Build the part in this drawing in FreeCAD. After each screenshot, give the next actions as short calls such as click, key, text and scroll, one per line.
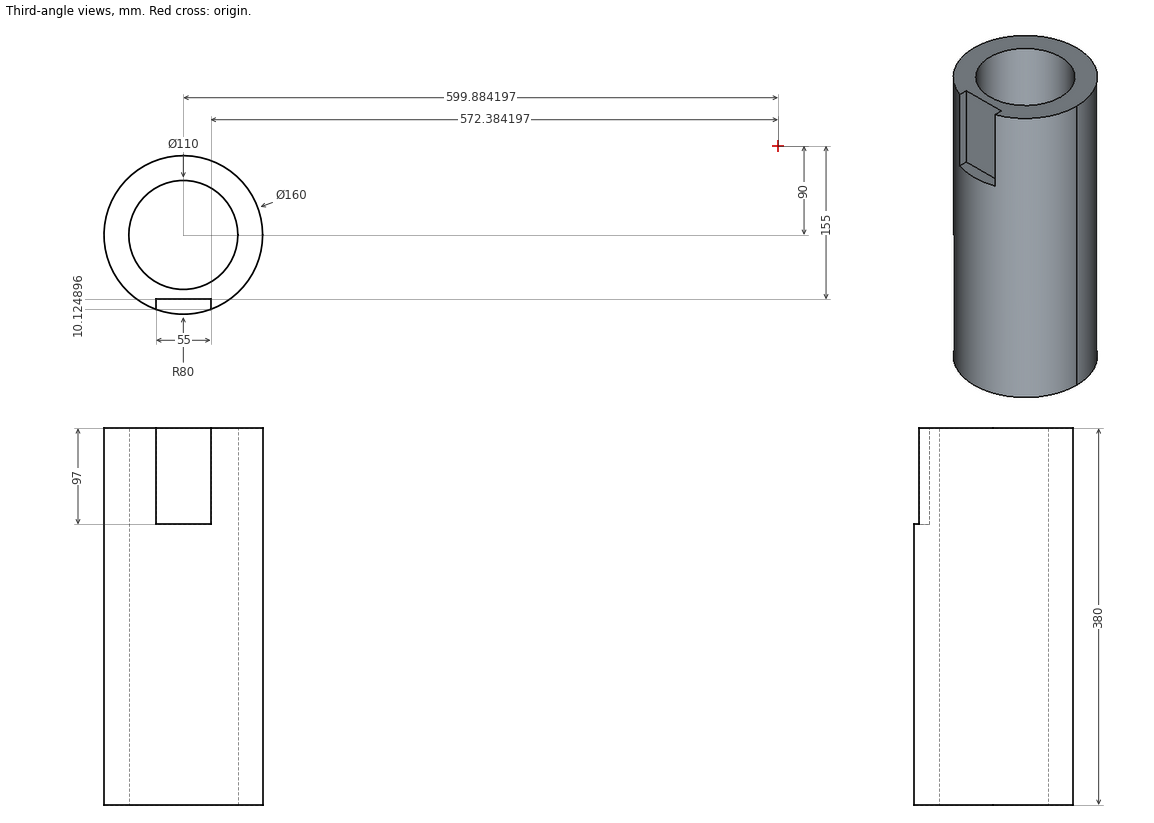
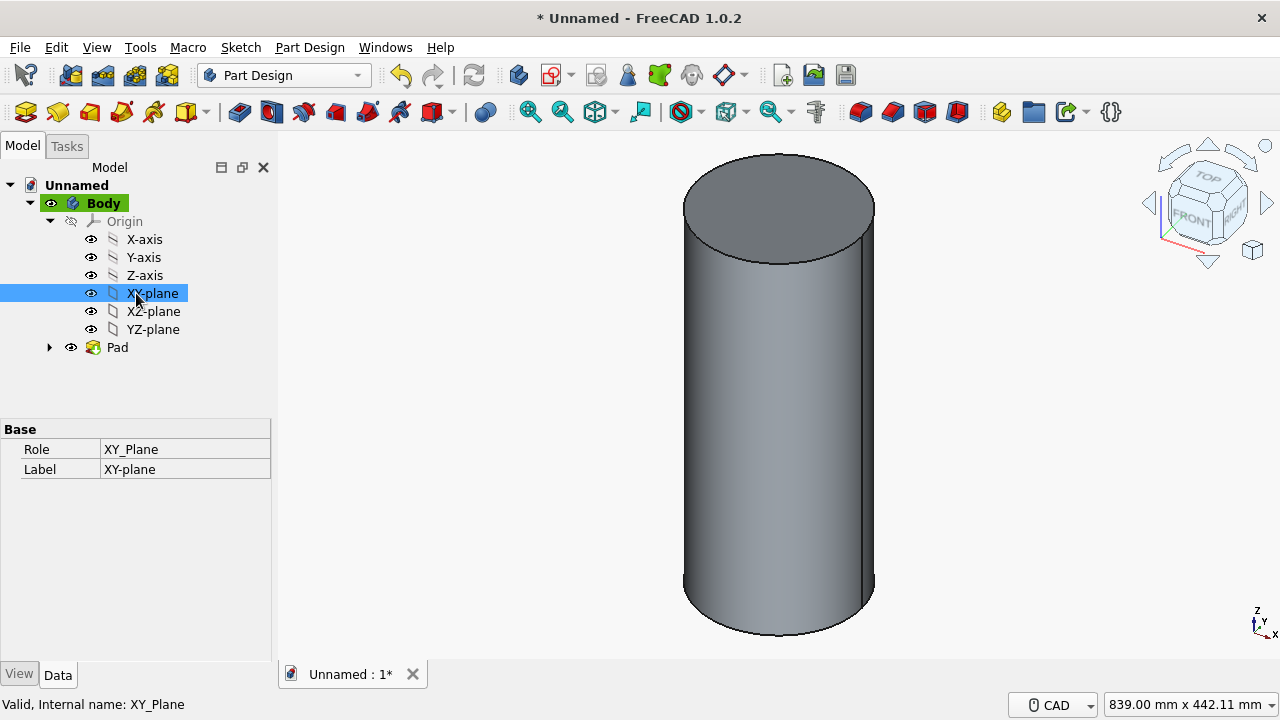
click(724, 76)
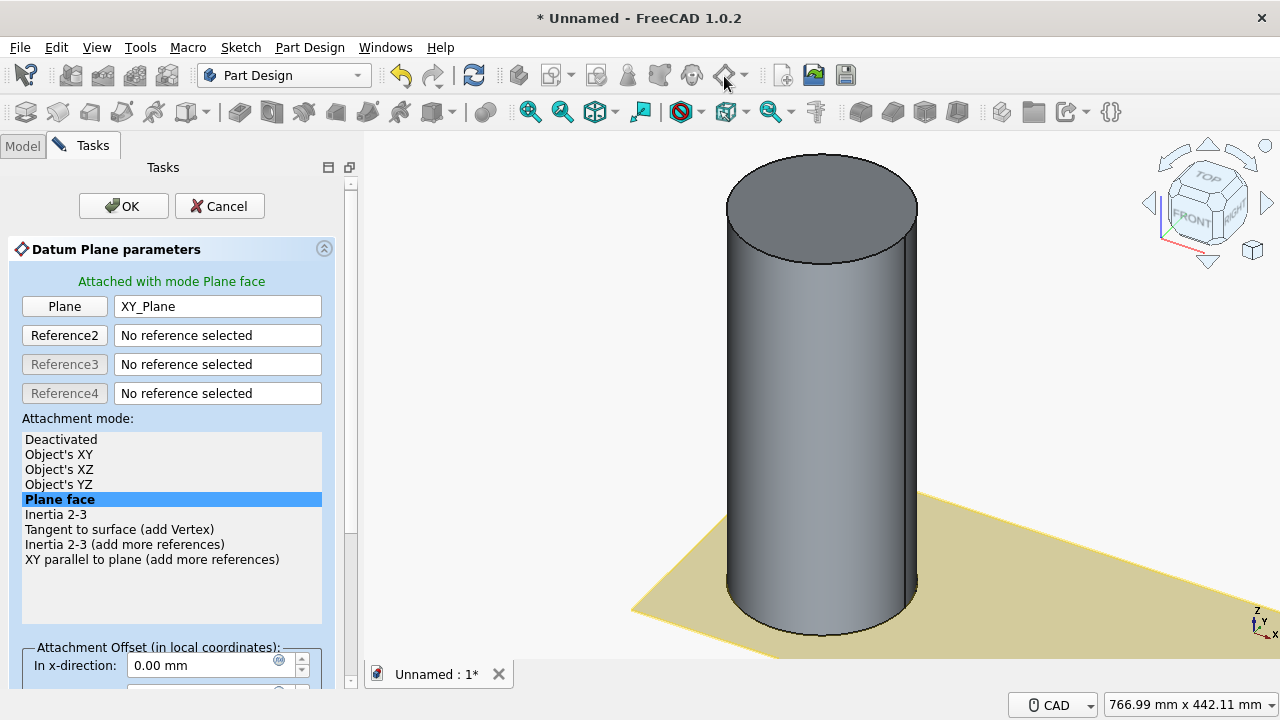
scroll(351, 432, down, 2)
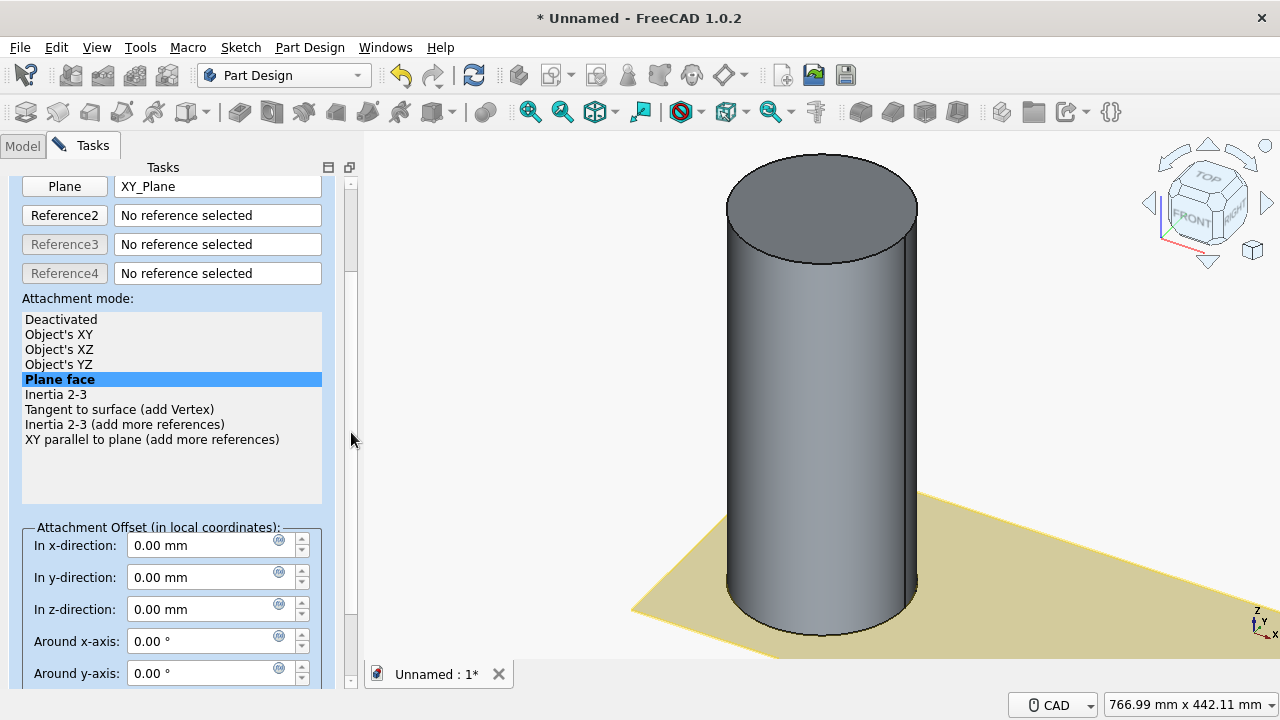
triple_click(210, 609)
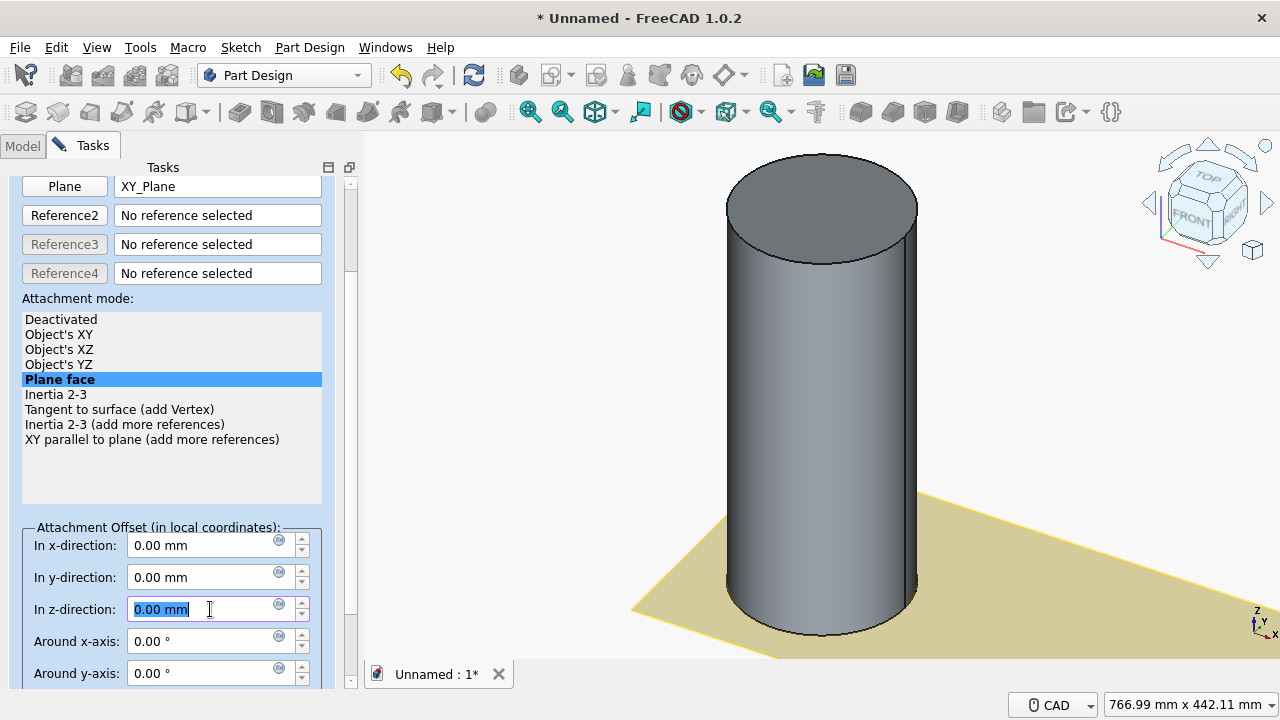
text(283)
key(Tab)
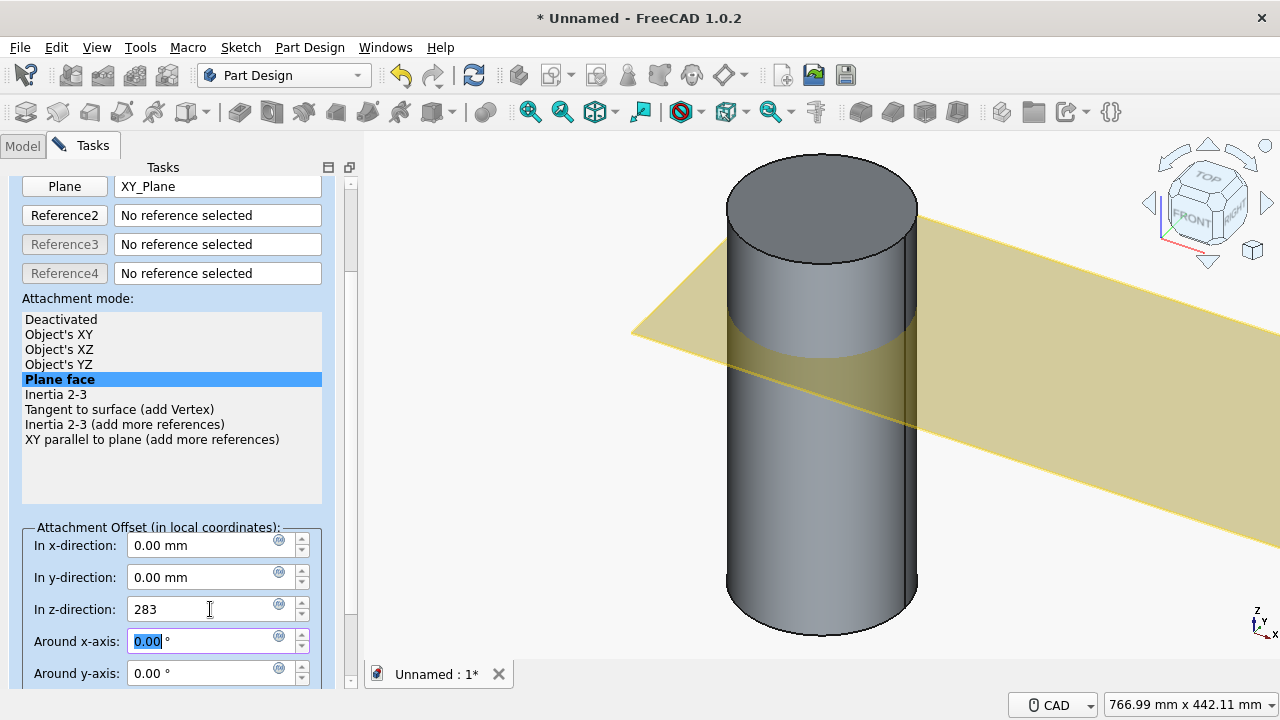
scroll(351, 432, up, 3)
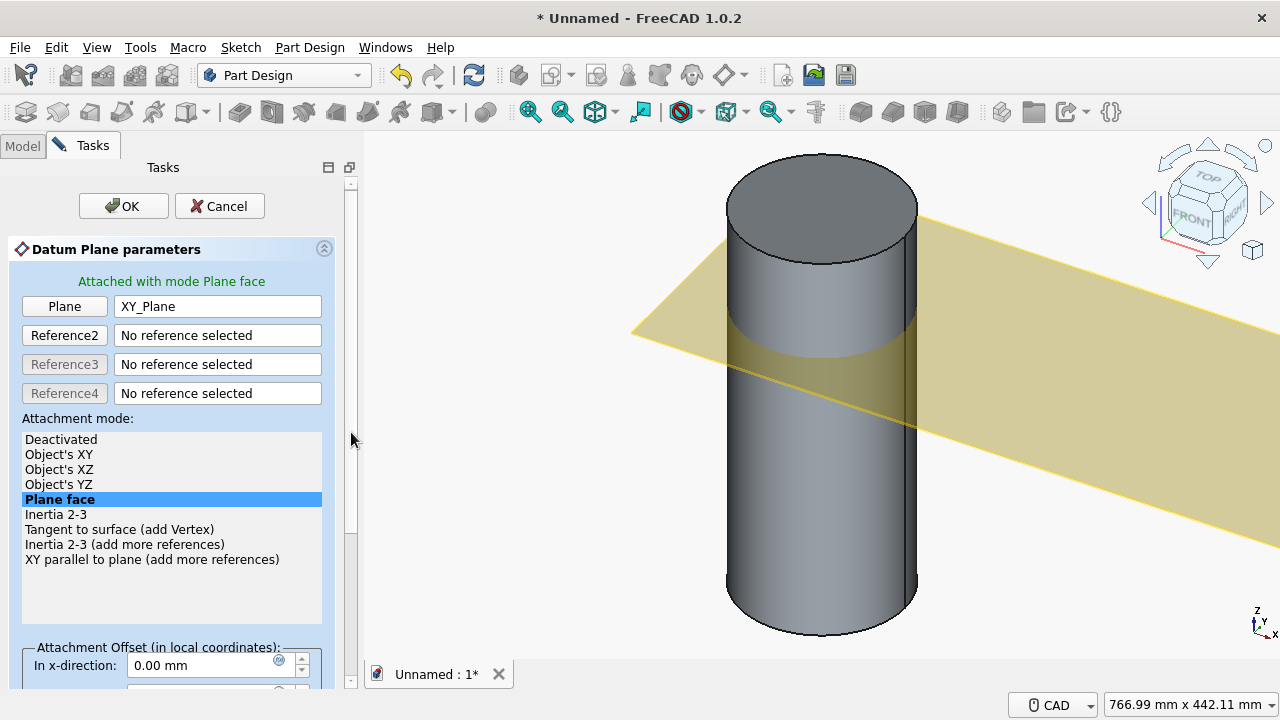
click(124, 206)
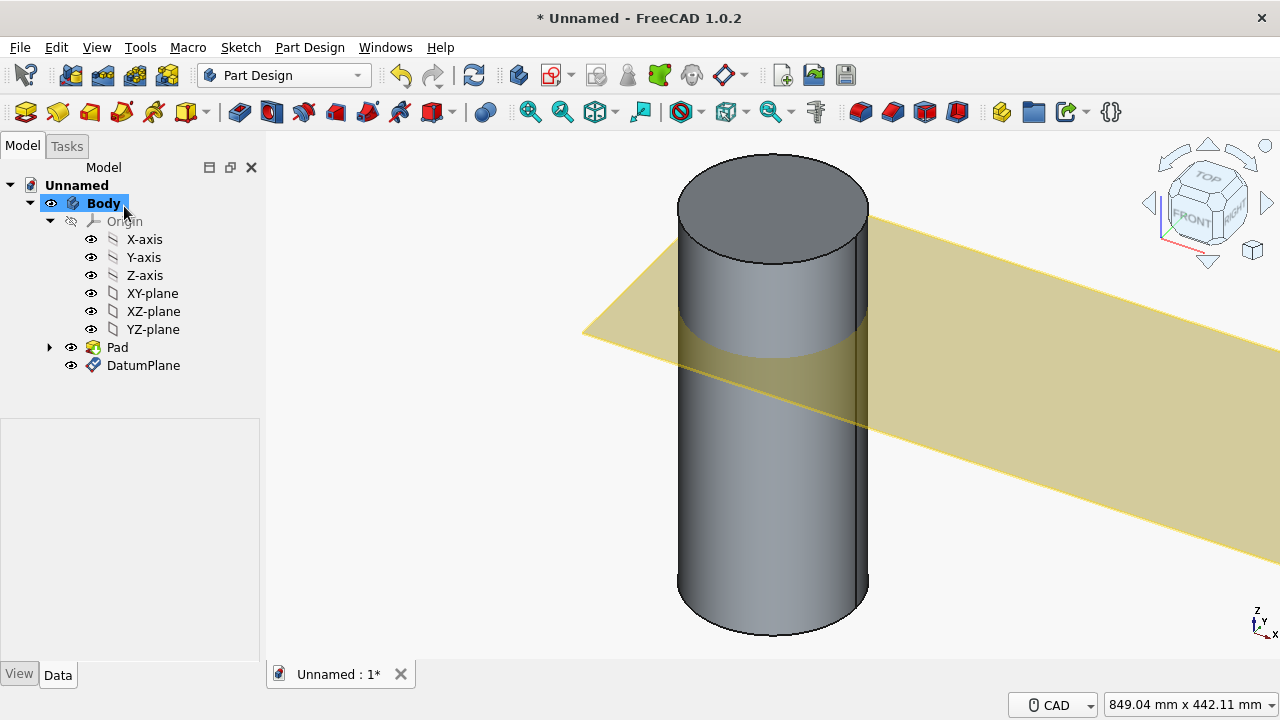
click(116, 365)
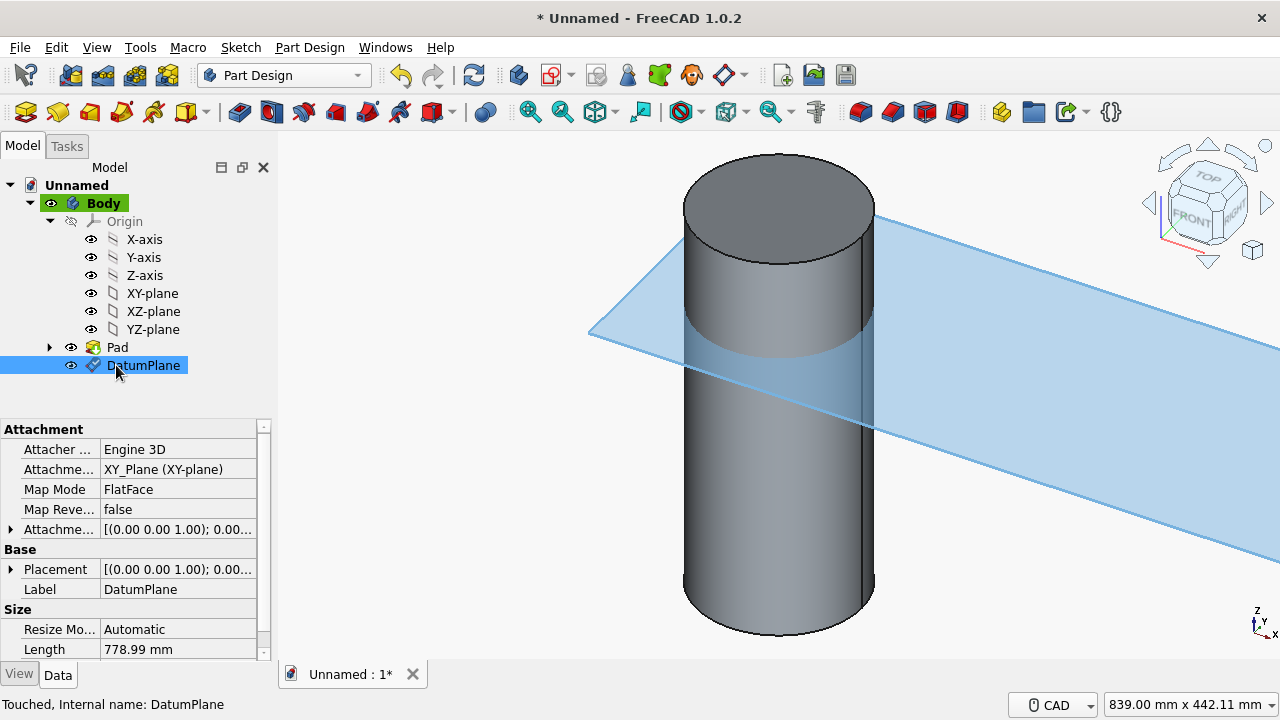
click(552, 76)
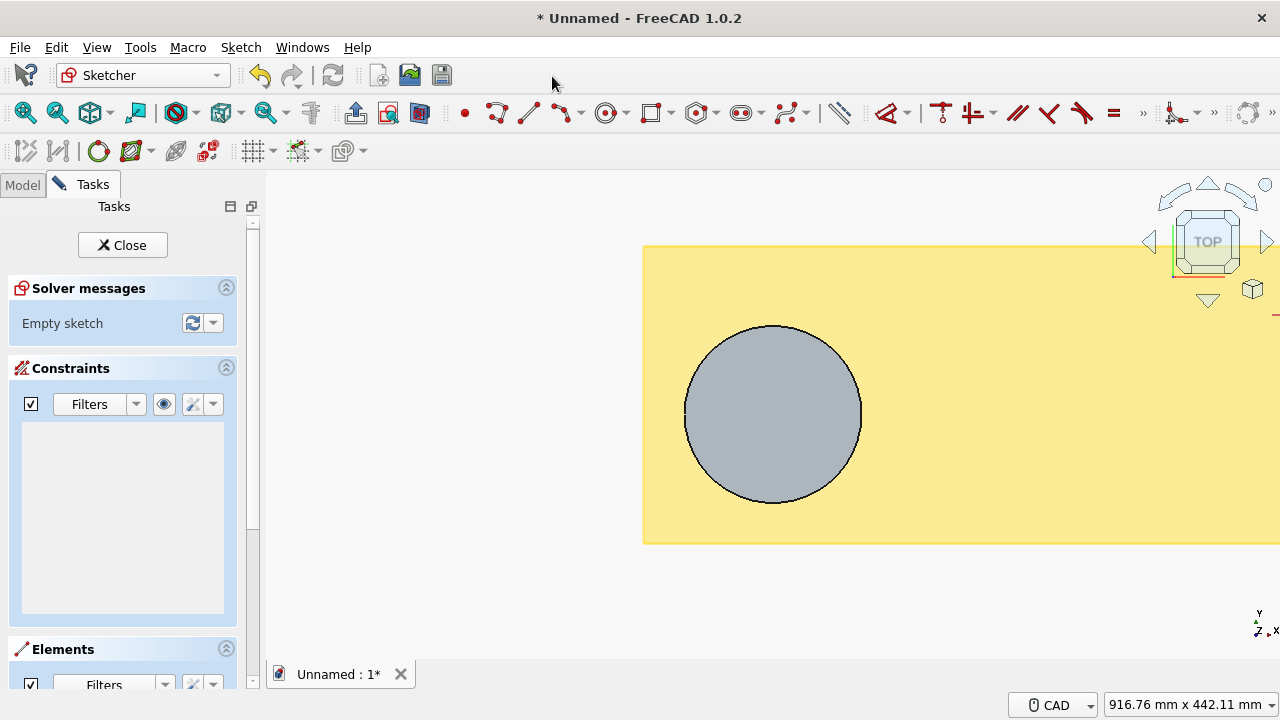
click(420, 114)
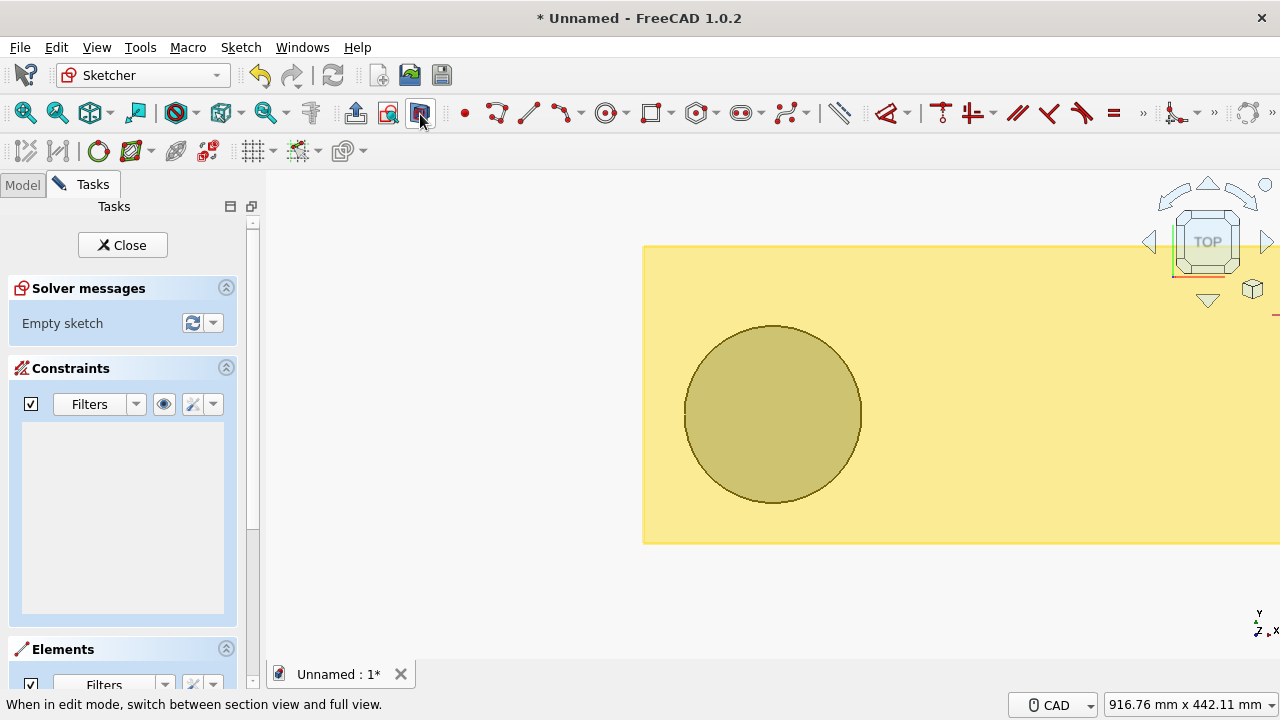
scroll(782, 505, up, 11)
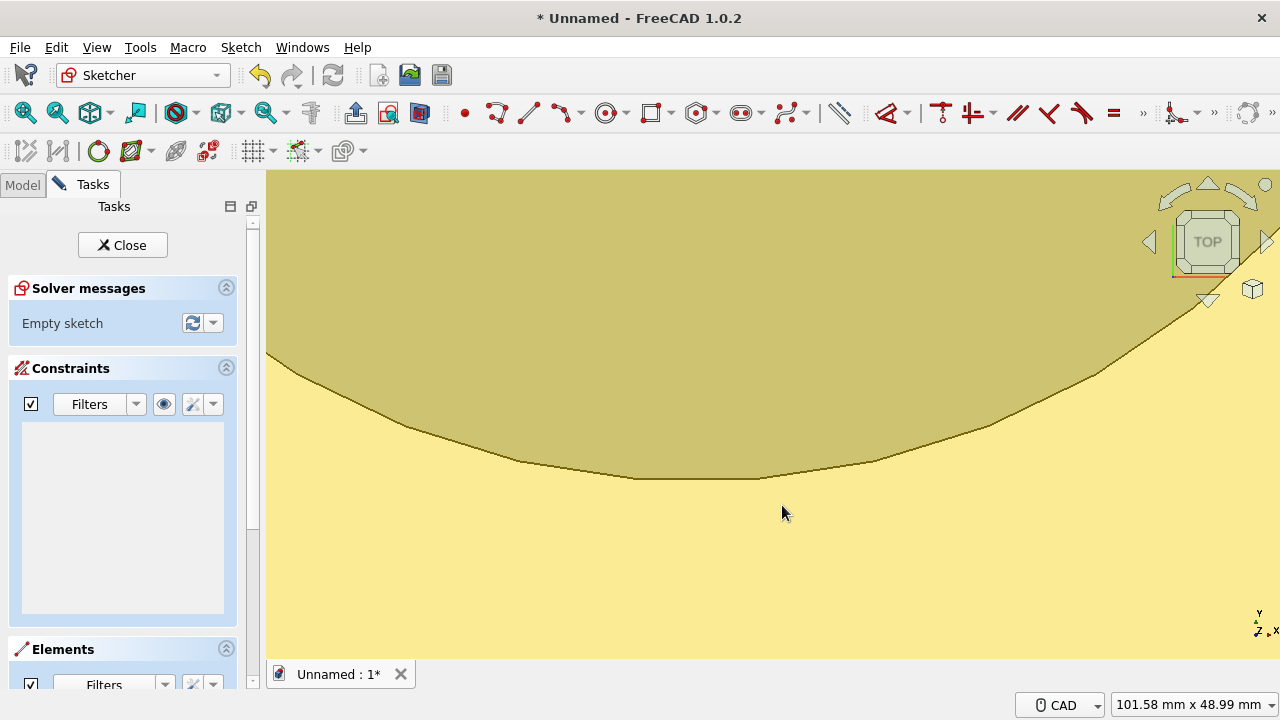
click(498, 114)